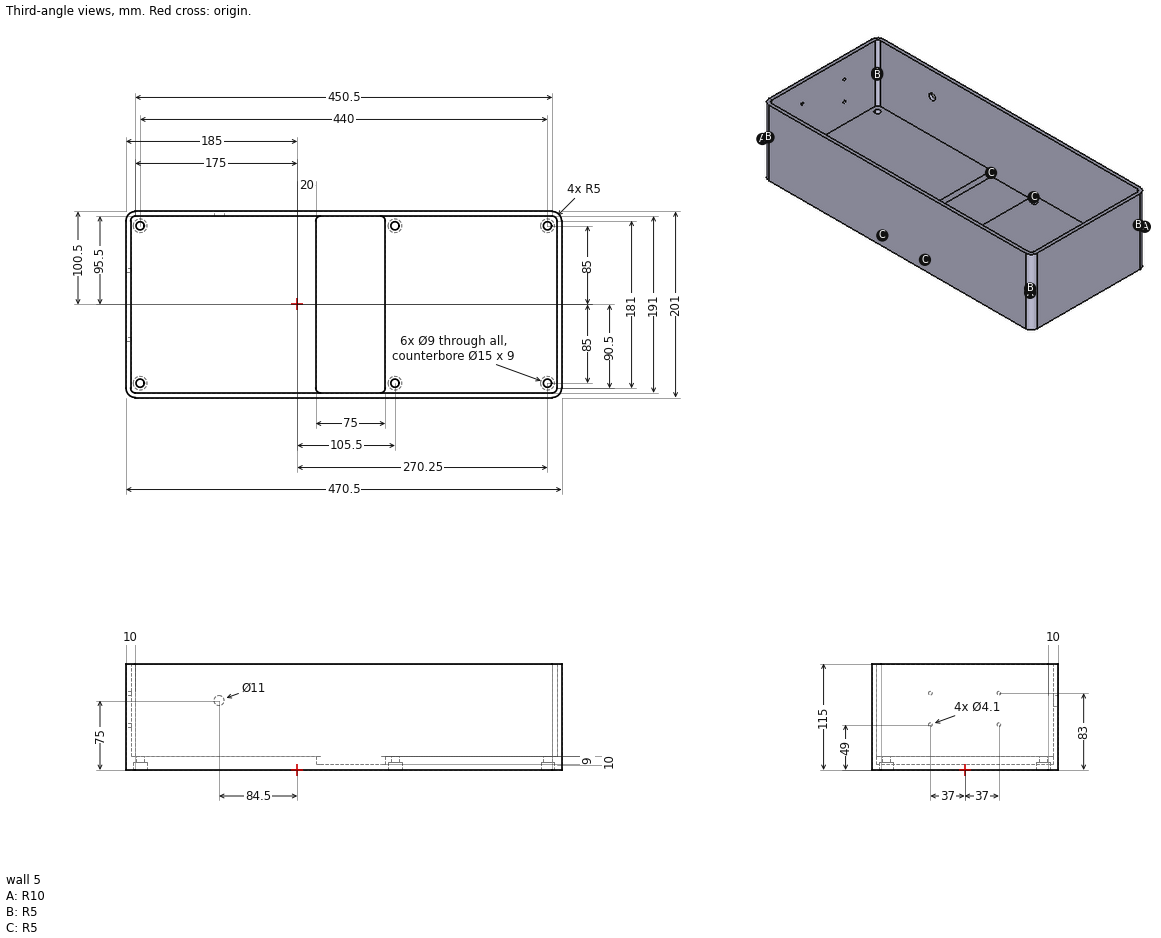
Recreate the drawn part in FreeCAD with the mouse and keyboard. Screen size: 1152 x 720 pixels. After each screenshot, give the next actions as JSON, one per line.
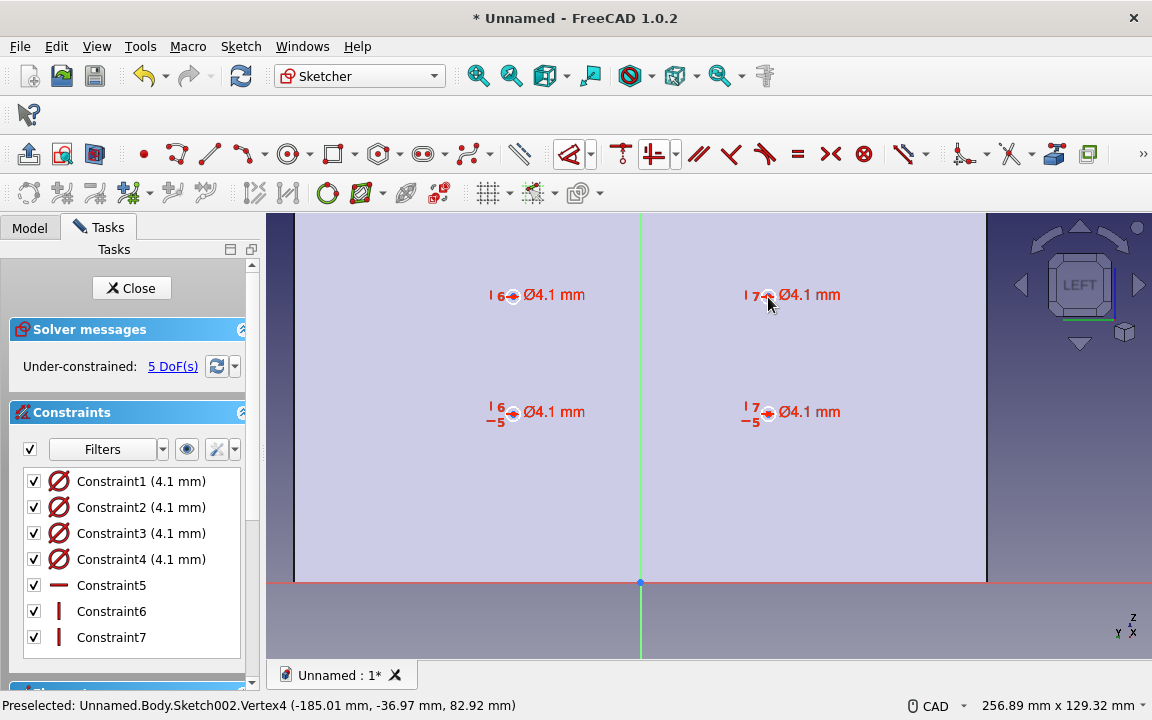
{"action": "left_click", "coordinate": [513, 297]}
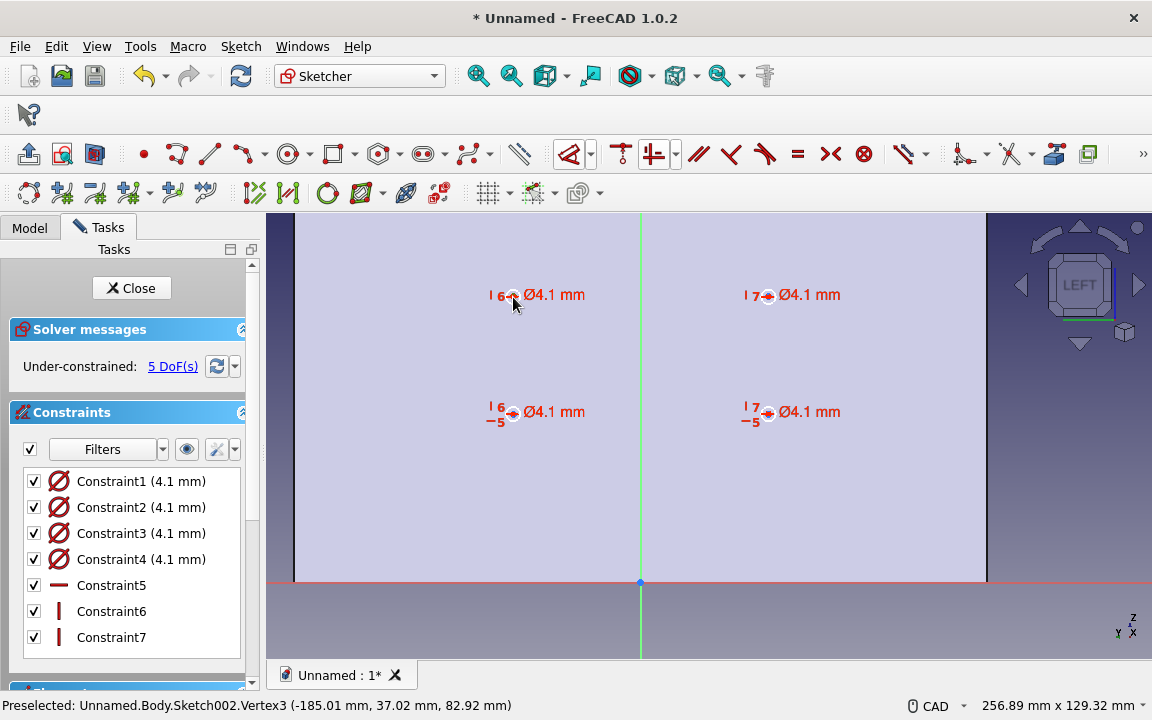
{"action": "left_click", "coordinate": [768, 297]}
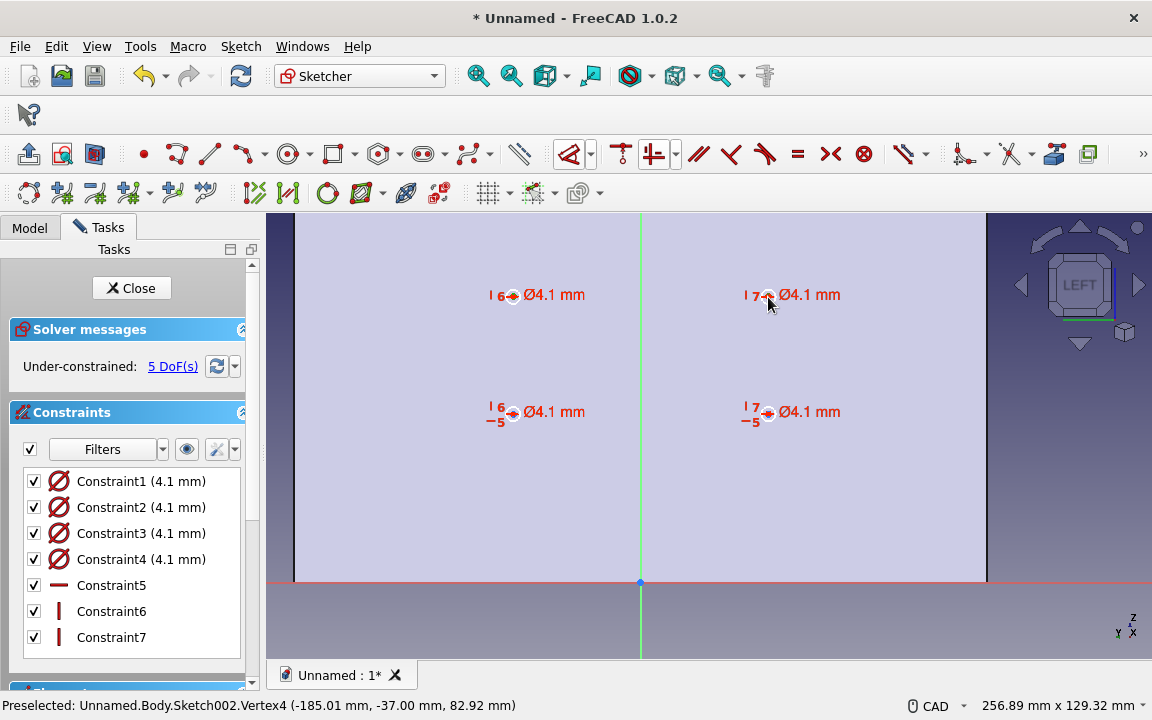
{"action": "left_click", "coordinate": [676, 154]}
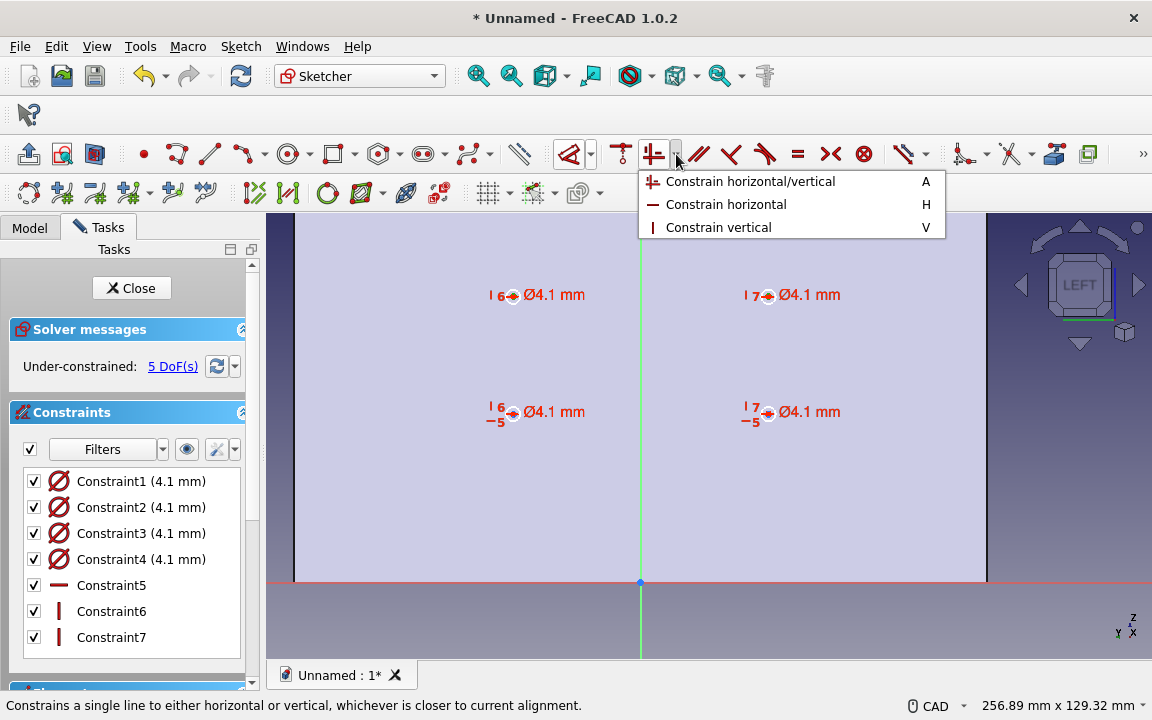
{"action": "left_click", "coordinate": [792, 204]}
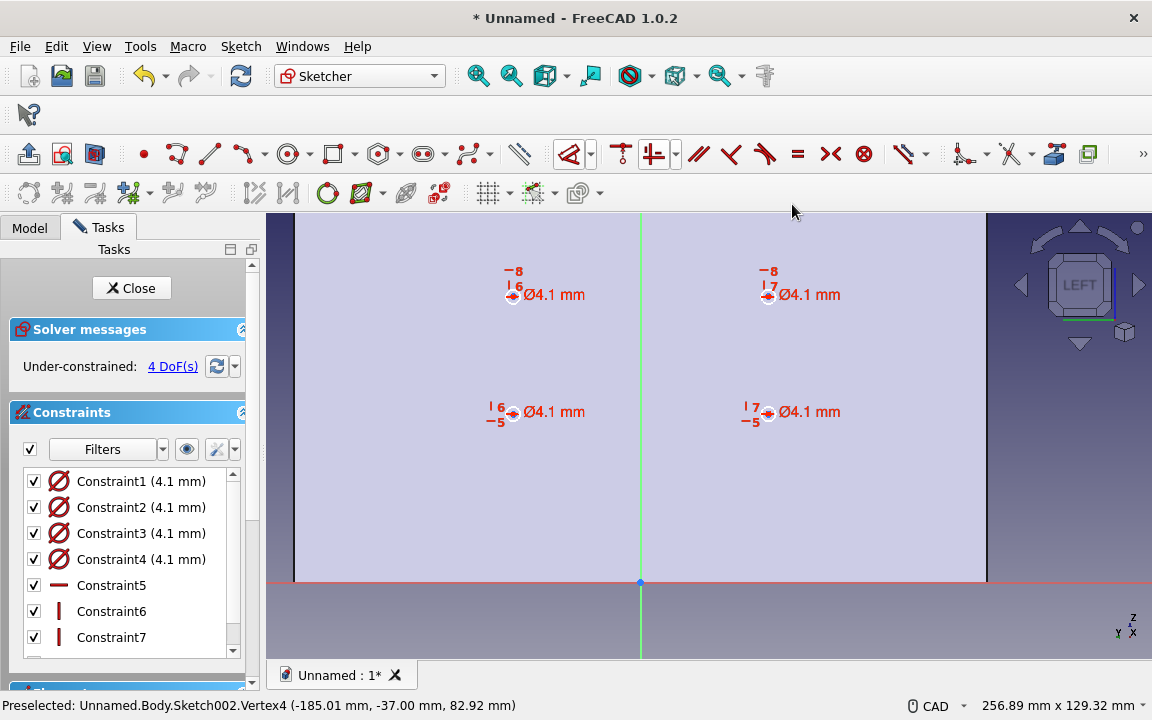
{"action": "key", "text": "d"}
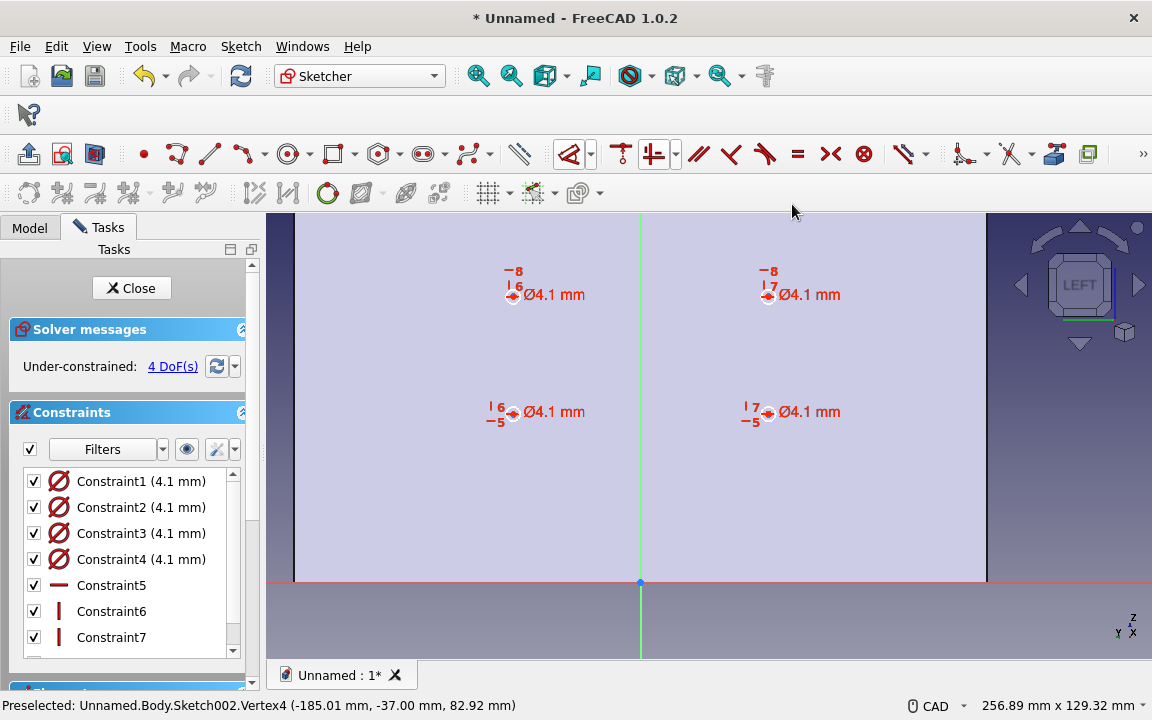
{"action": "left_click", "coordinate": [768, 414]}
{"action": "left_click", "coordinate": [705, 617]}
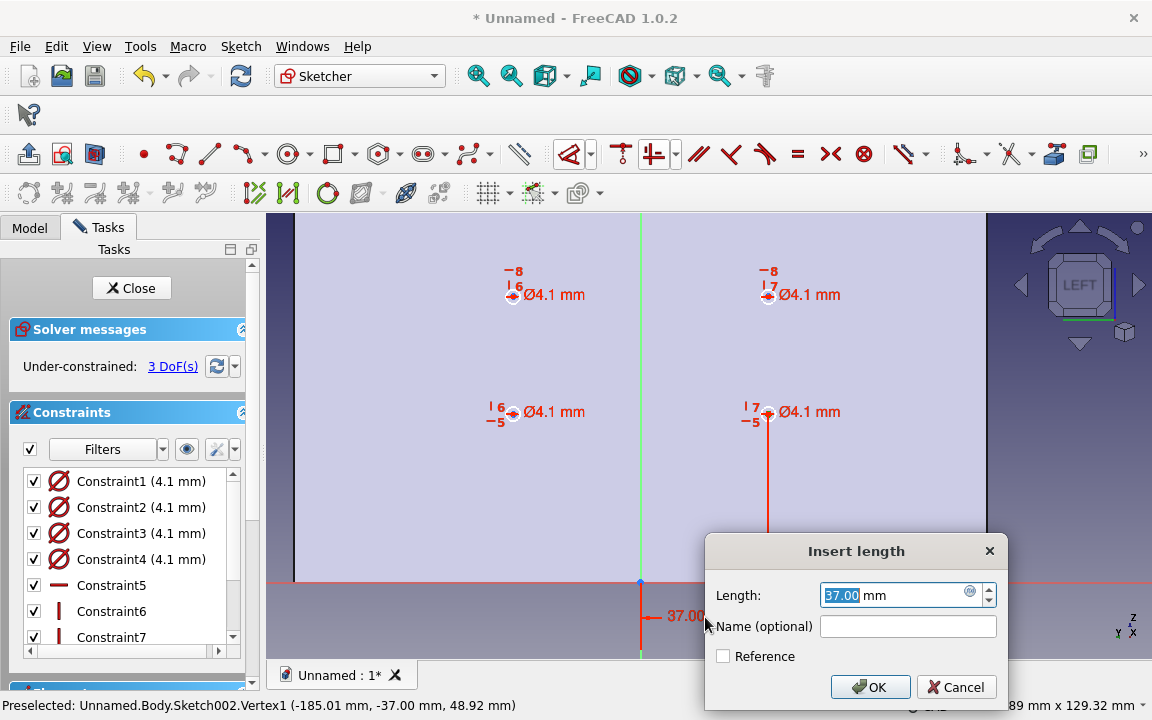
{"action": "type", "text": "37"}
{"action": "key", "text": "Return"}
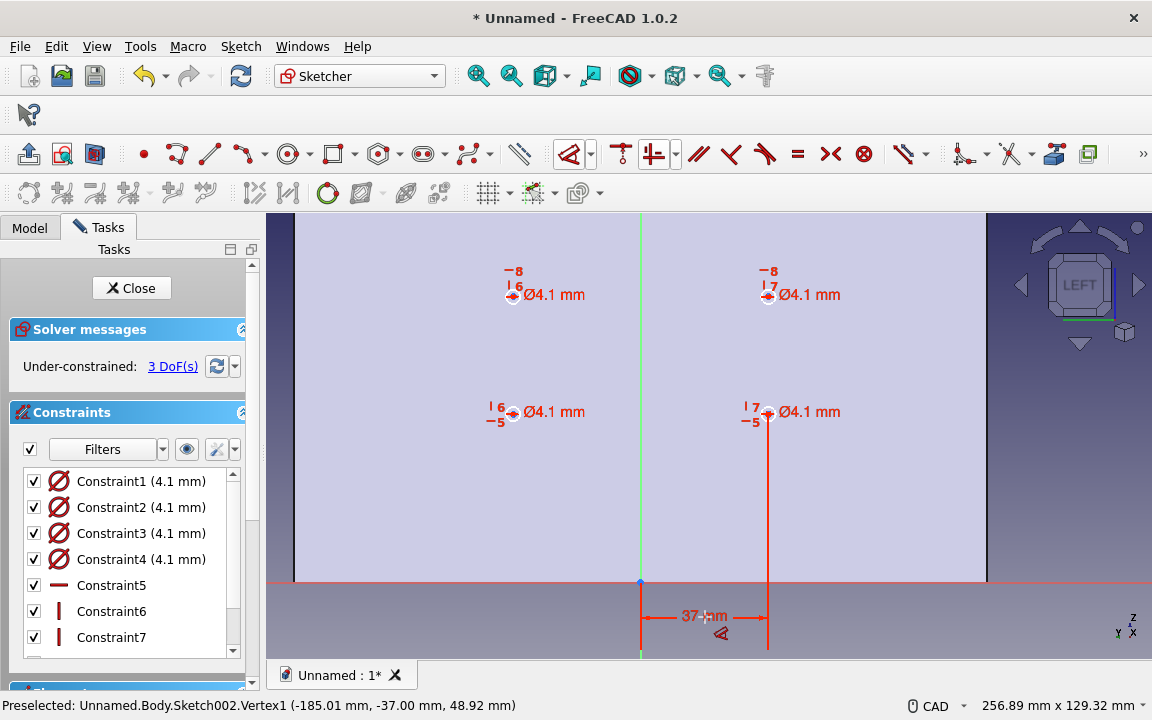
{"action": "left_click", "coordinate": [768, 414]}
{"action": "left_click", "coordinate": [802, 498]}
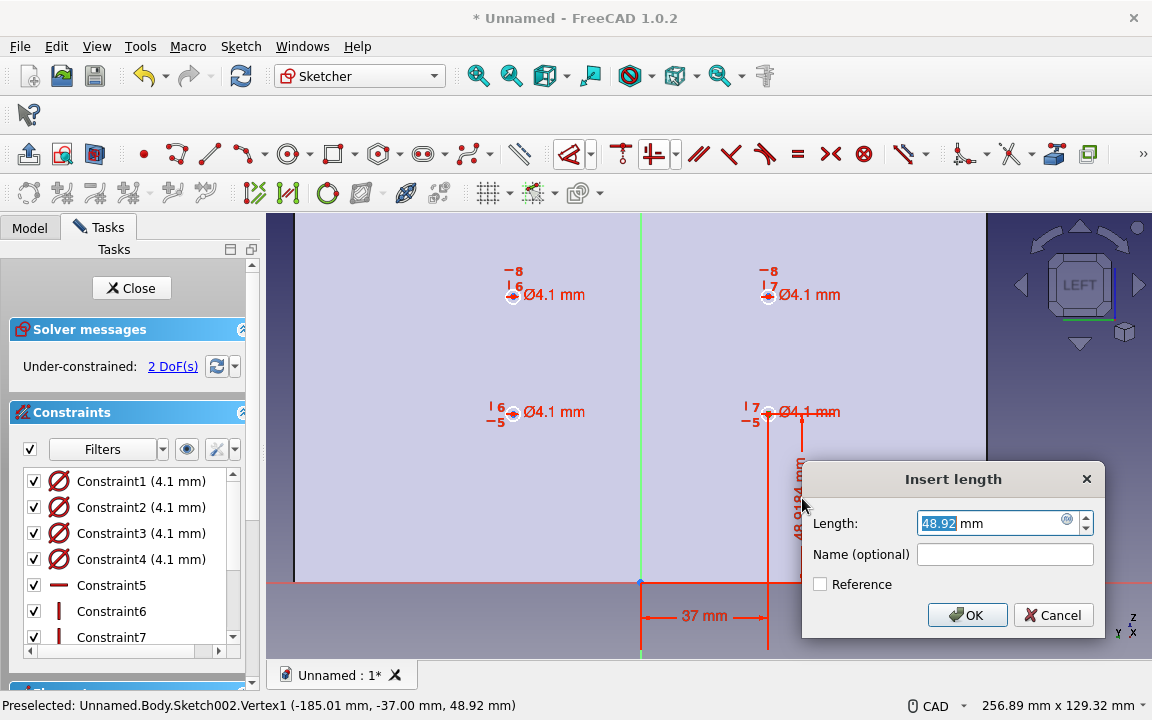
{"action": "type", "text": "49"}
{"action": "key", "text": "Return"}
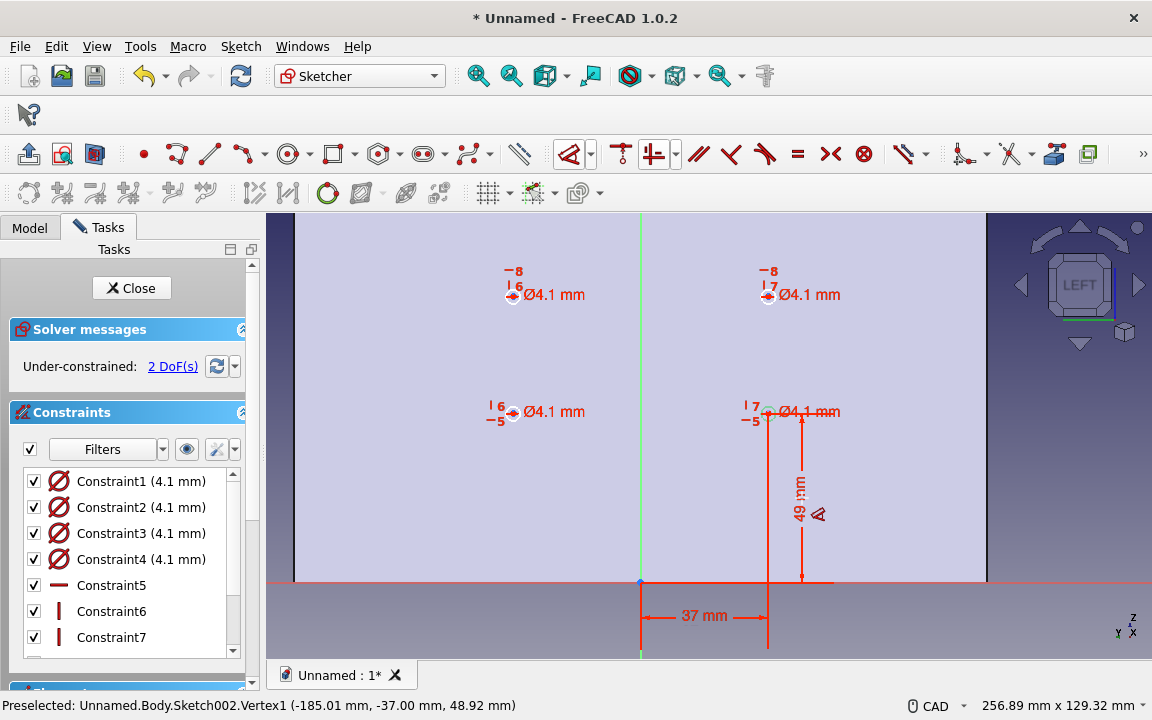
{"action": "left_click", "coordinate": [513, 414]}
{"action": "left_click", "coordinate": [577, 617]}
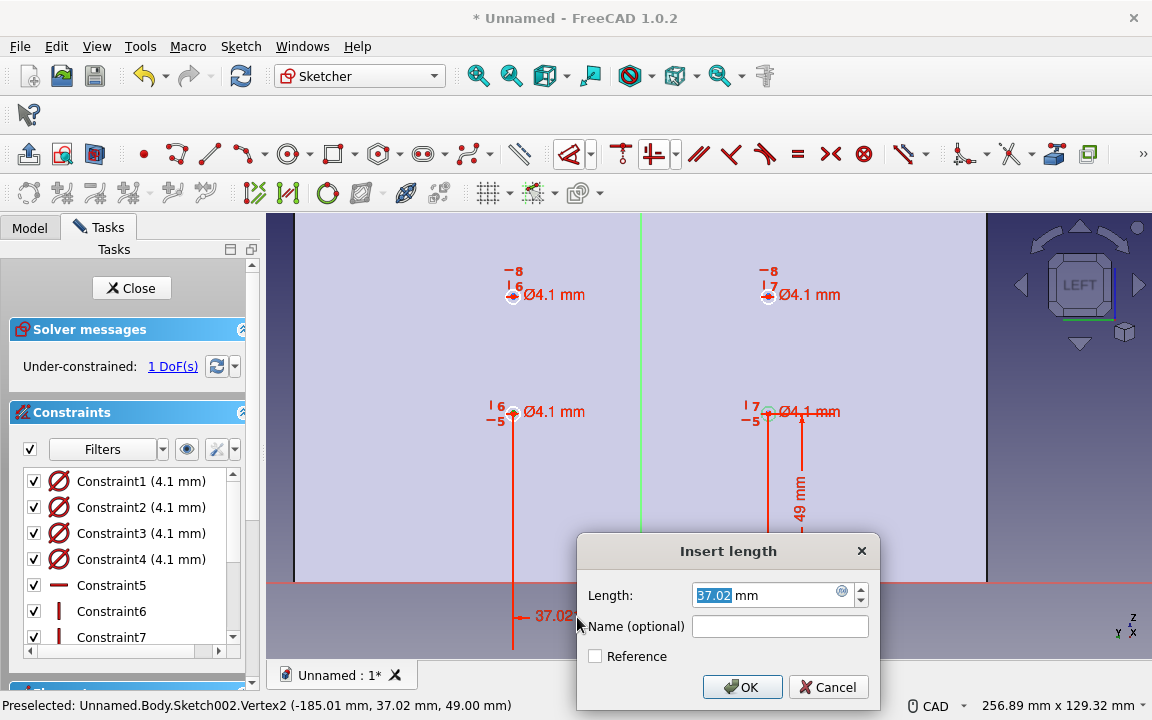
{"action": "type", "text": "37"}
{"action": "key", "text": "Return"}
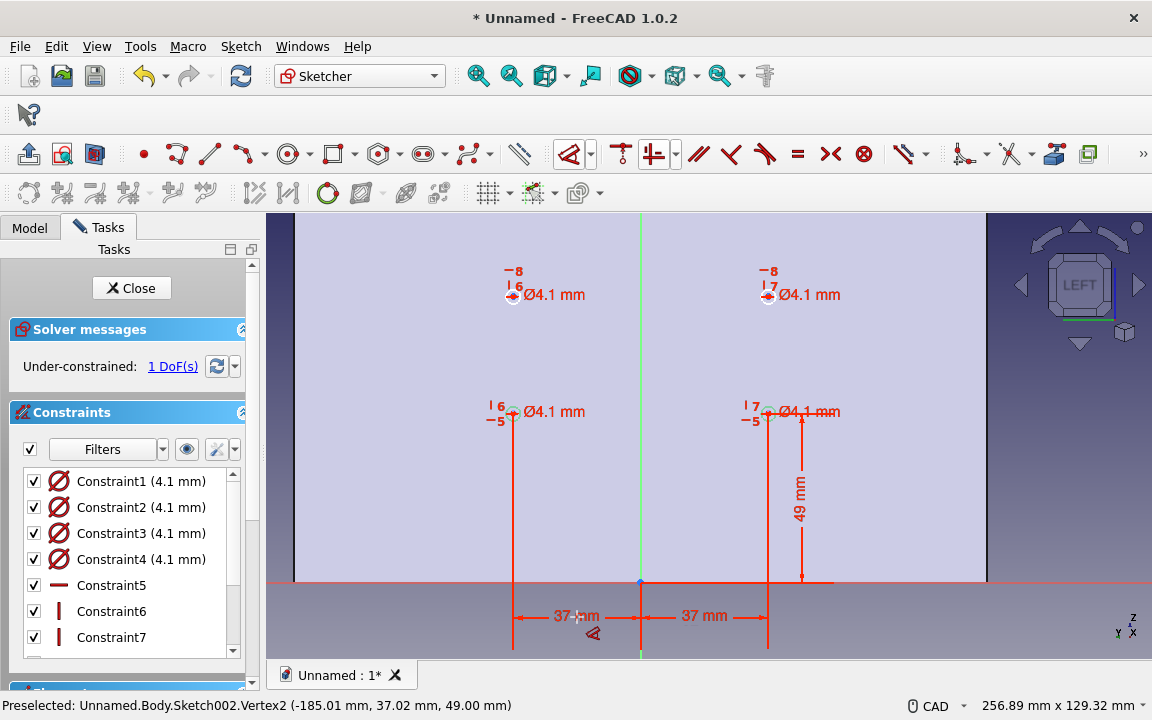
{"action": "left_click", "coordinate": [513, 297]}
{"action": "left_click", "coordinate": [479, 440]}